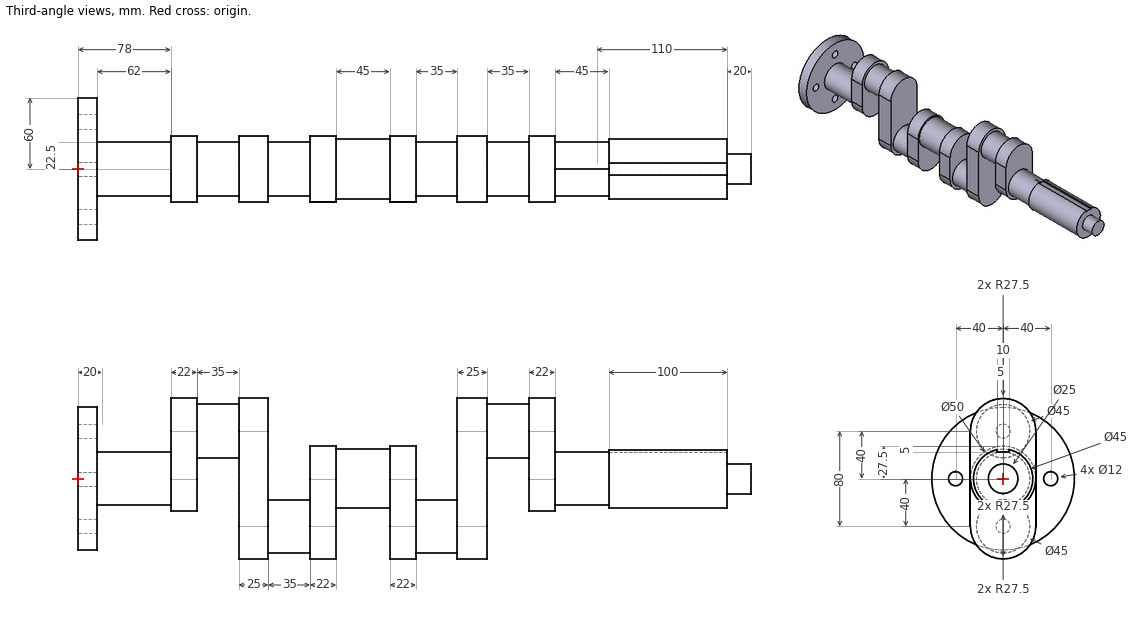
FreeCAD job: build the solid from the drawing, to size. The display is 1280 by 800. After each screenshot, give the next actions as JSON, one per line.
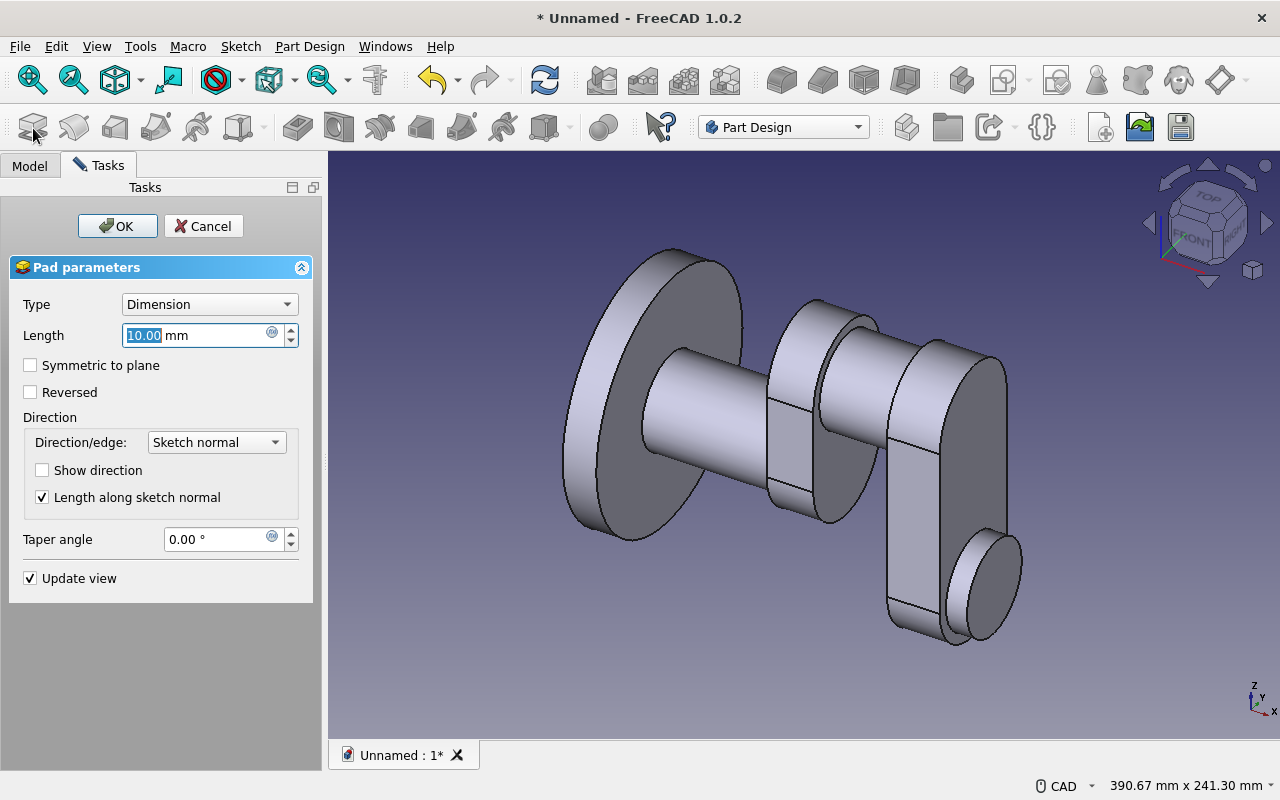
{"action": "type", "text": "35"}
{"action": "key", "text": "Tab"}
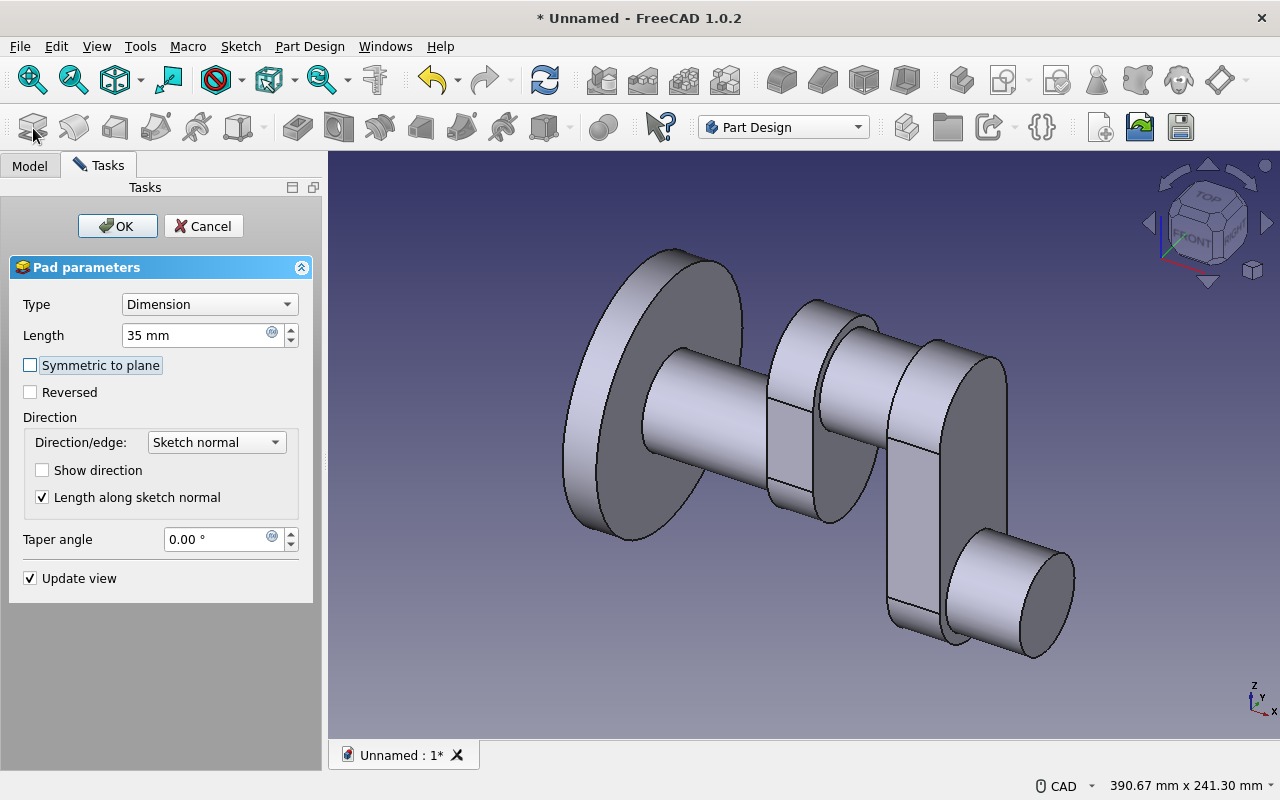
{"action": "left_click", "coordinate": [118, 226]}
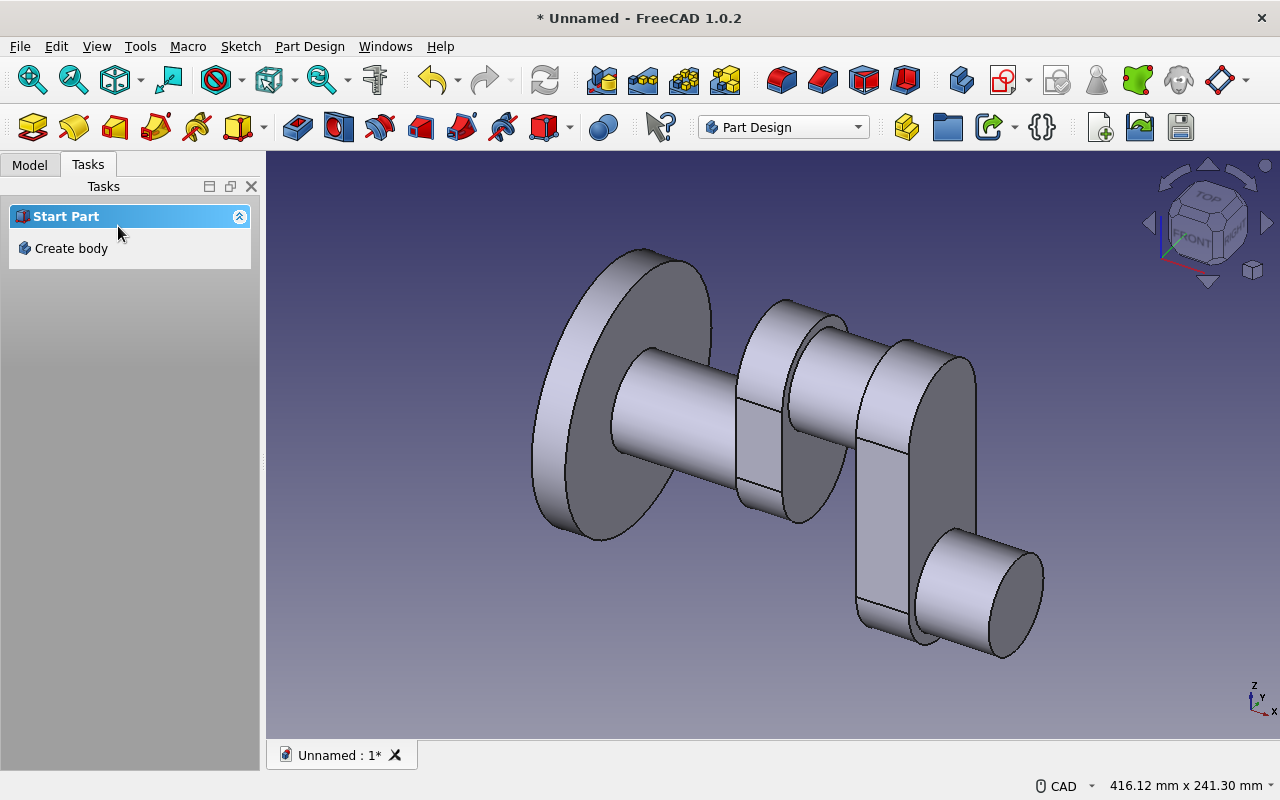
{"action": "left_click", "coordinate": [1016, 604]}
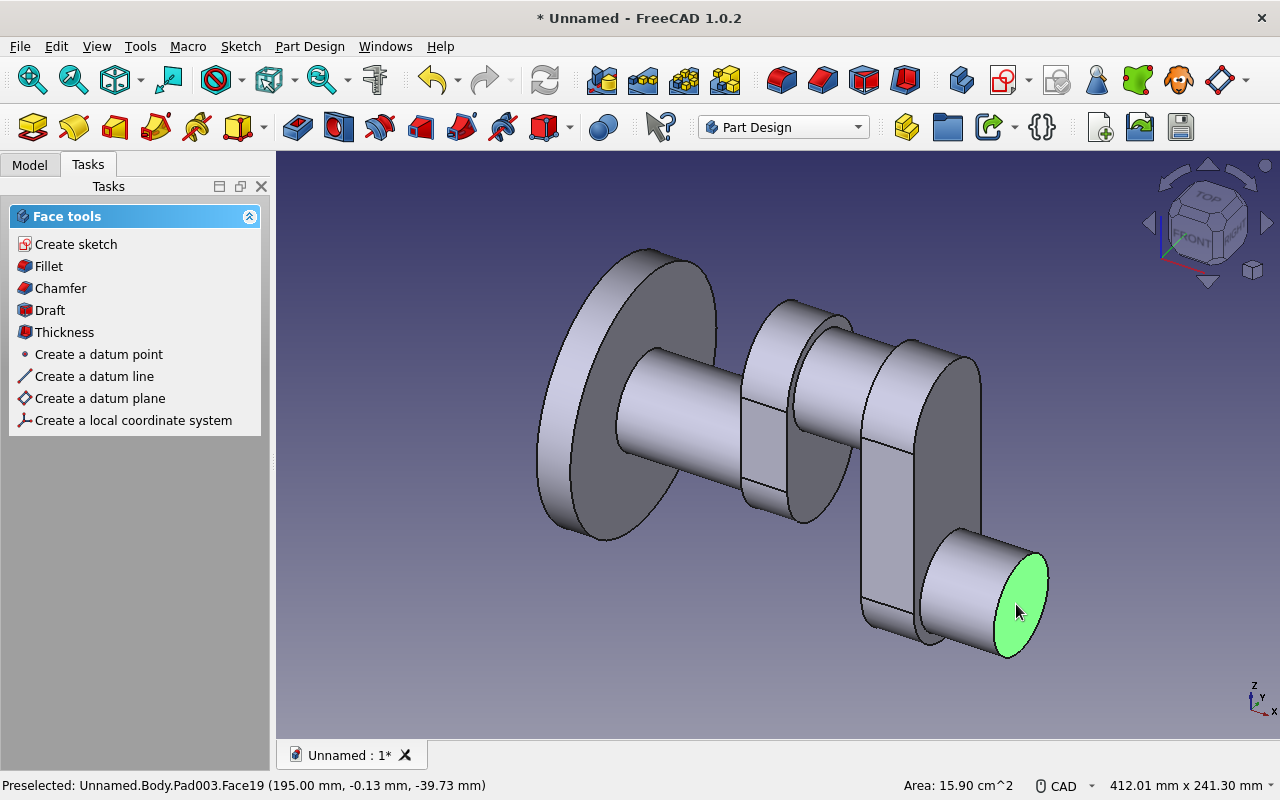
{"action": "left_click", "coordinate": [1002, 80]}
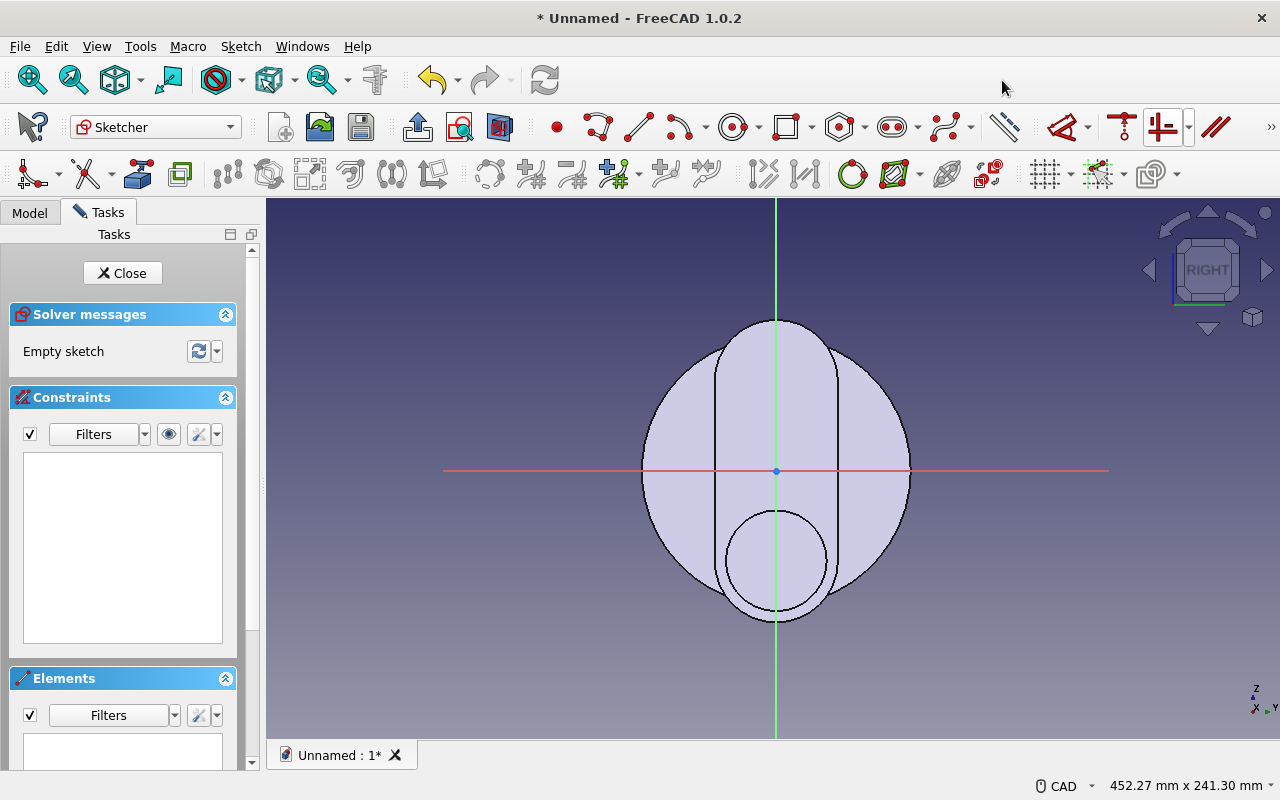
{"action": "scroll", "coordinate": [922, 613], "scroll_direction": "up", "scroll_amount": 2}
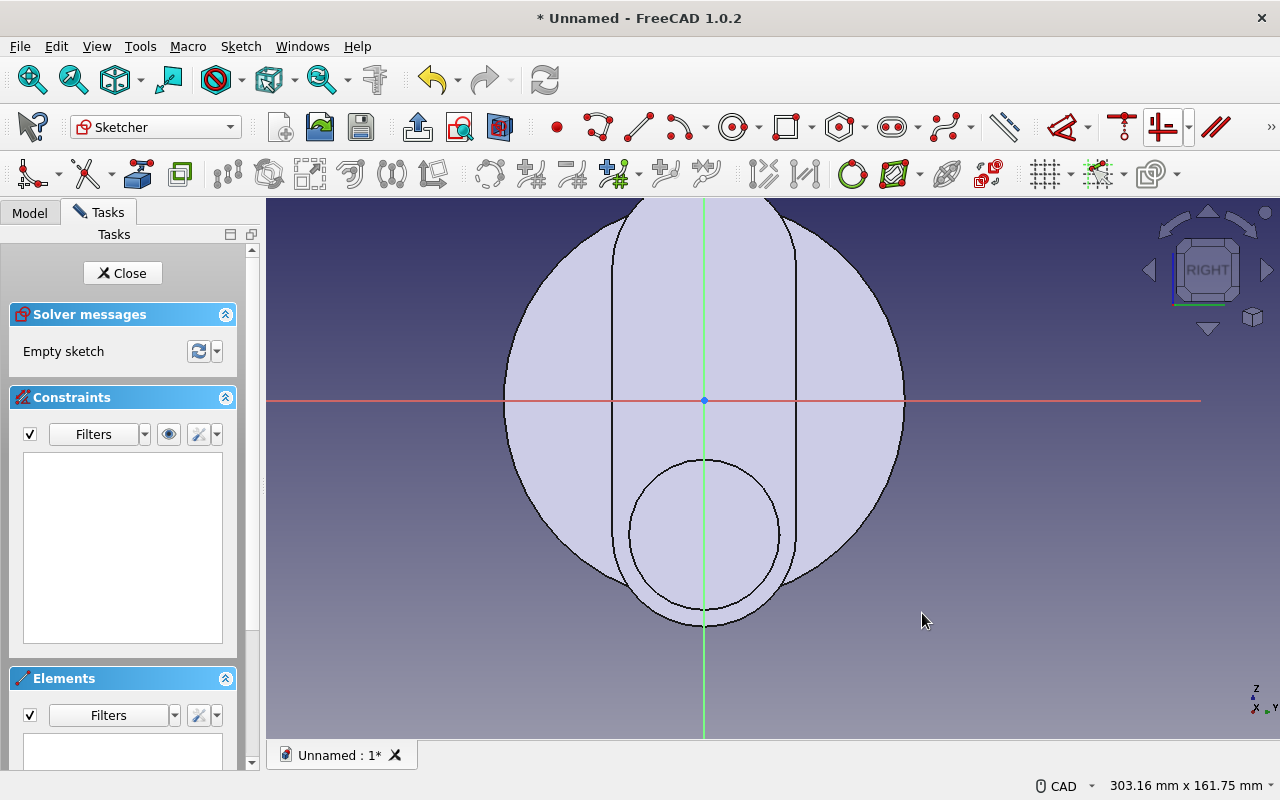
{"action": "left_click", "coordinate": [892, 128]}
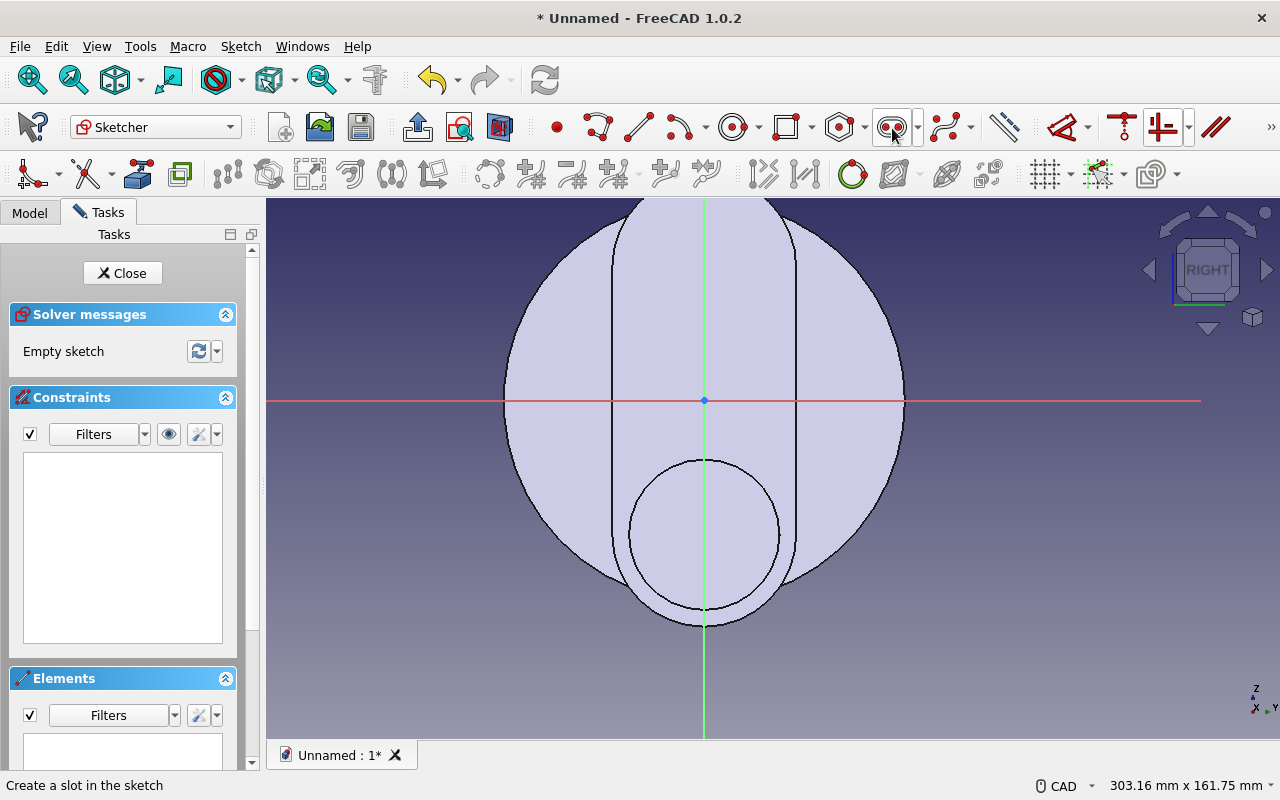
{"action": "left_click", "coordinate": [704, 401]}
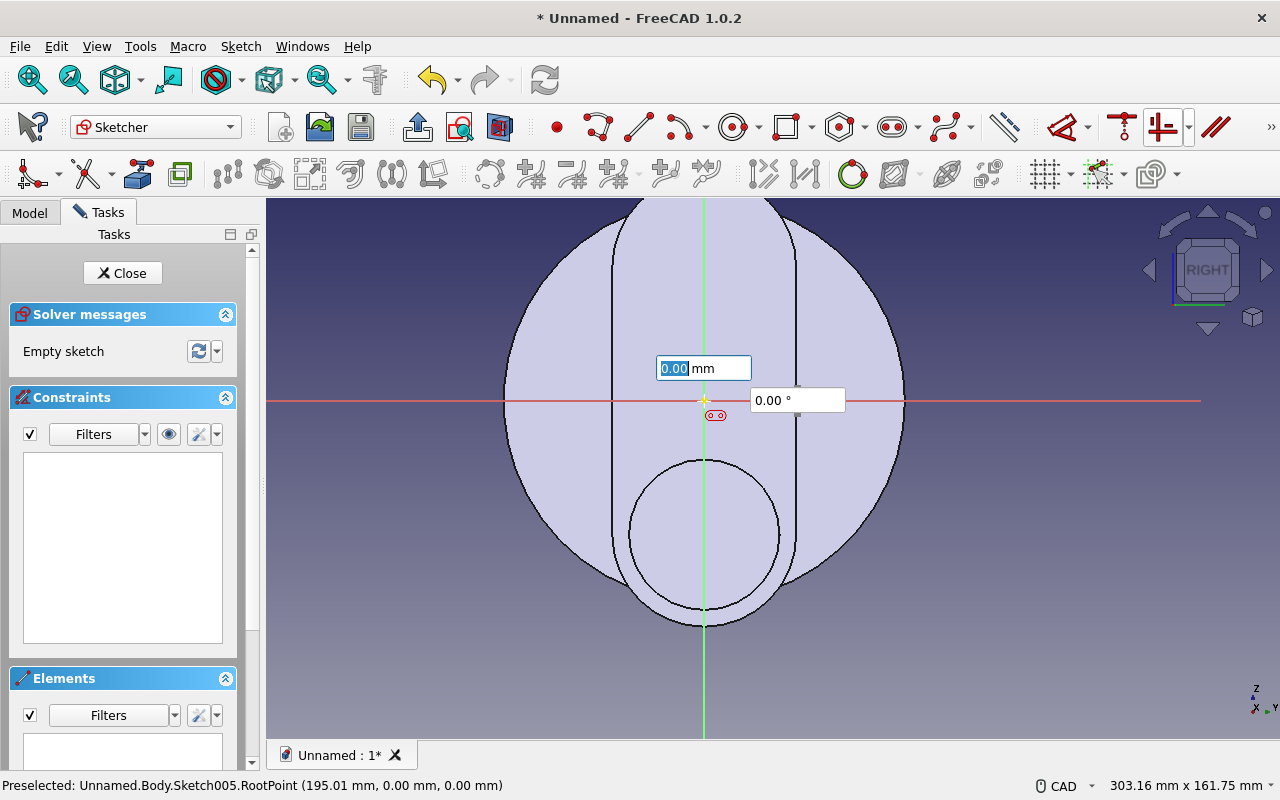
{"action": "left_click", "coordinate": [713, 535]}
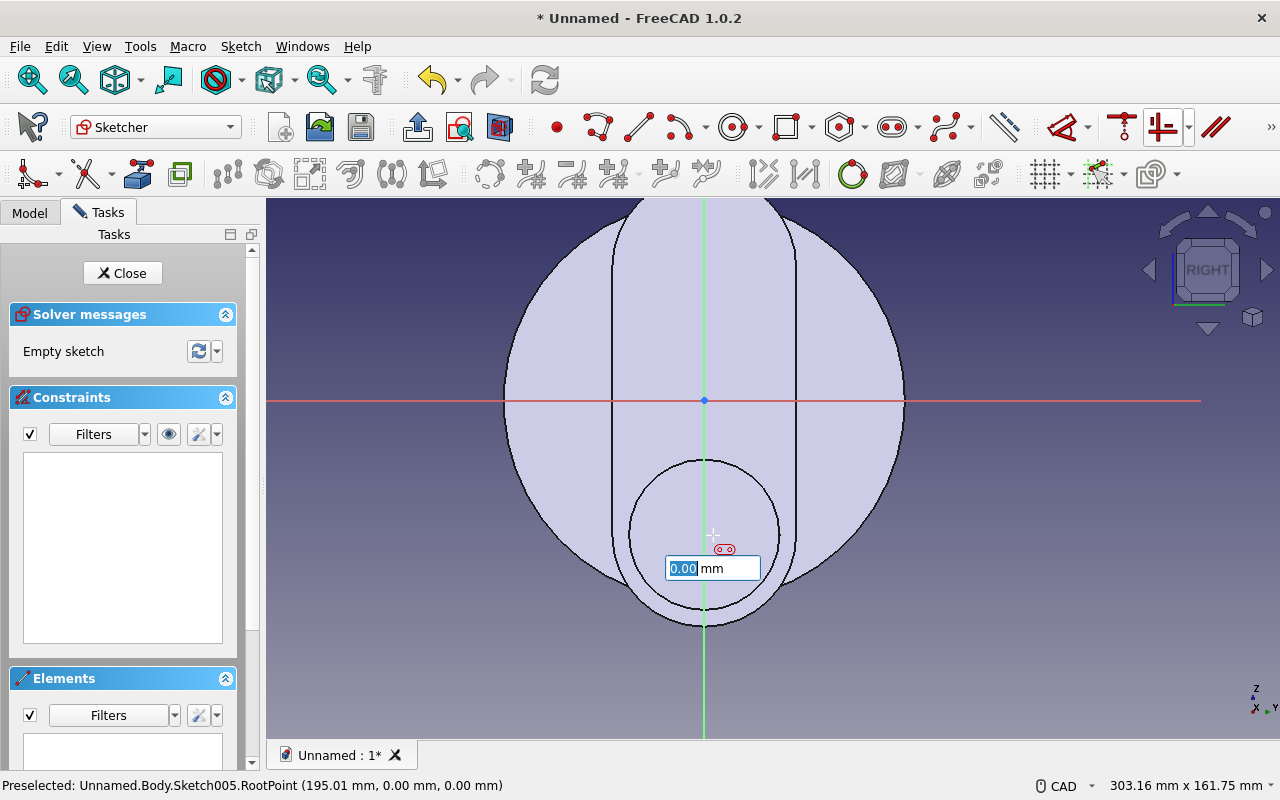
{"action": "left_click", "coordinate": [612, 468]}
{"action": "key", "text": "Escape"}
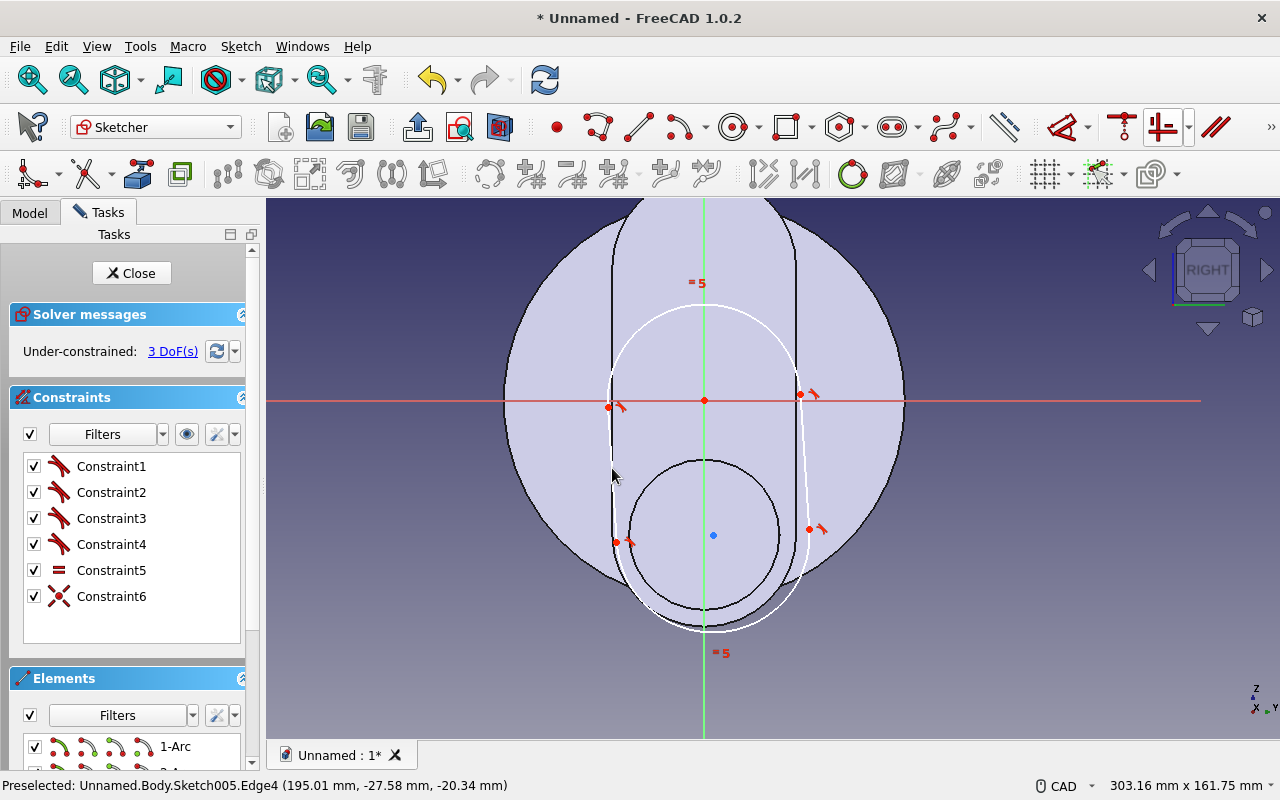
{"action": "left_click", "coordinate": [803, 435]}